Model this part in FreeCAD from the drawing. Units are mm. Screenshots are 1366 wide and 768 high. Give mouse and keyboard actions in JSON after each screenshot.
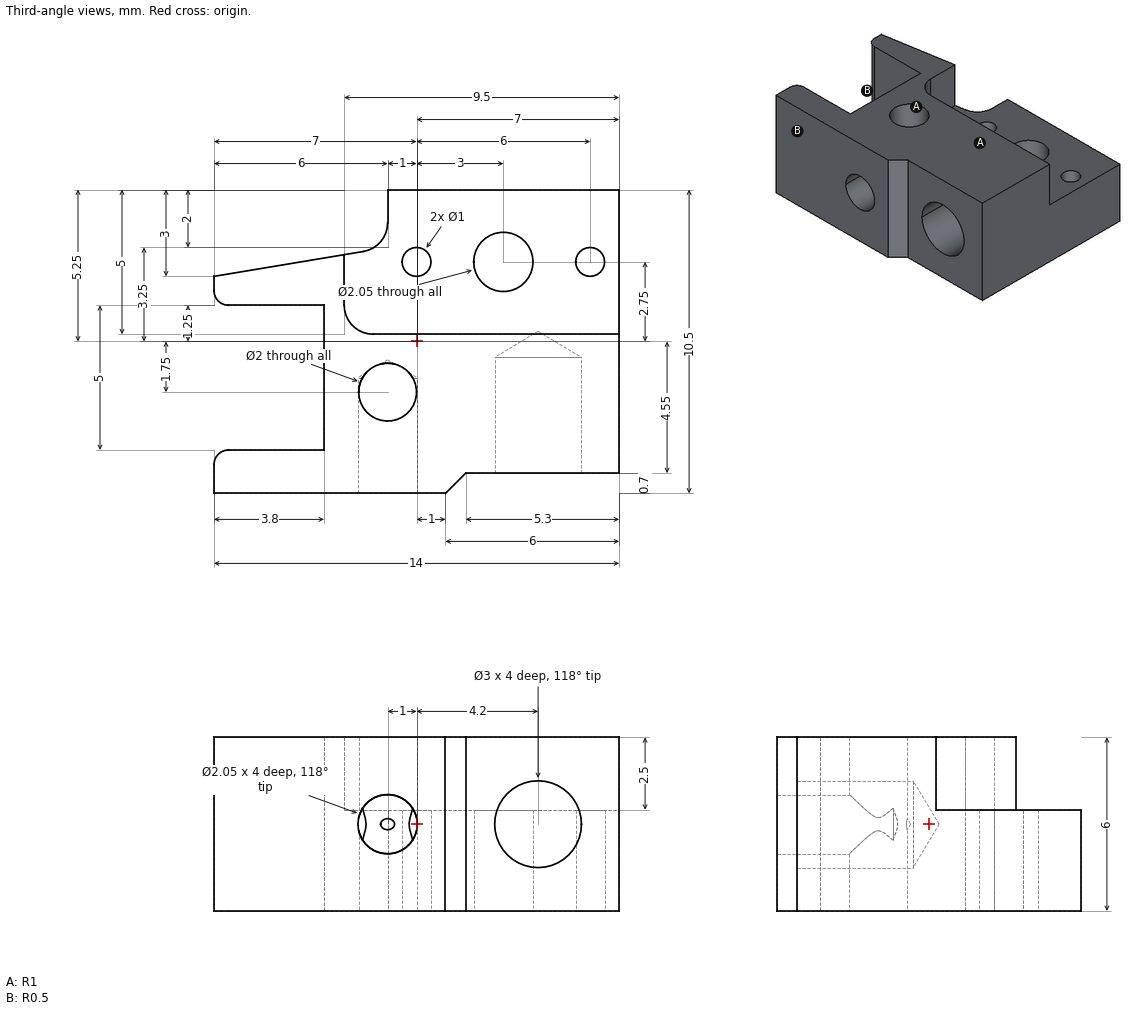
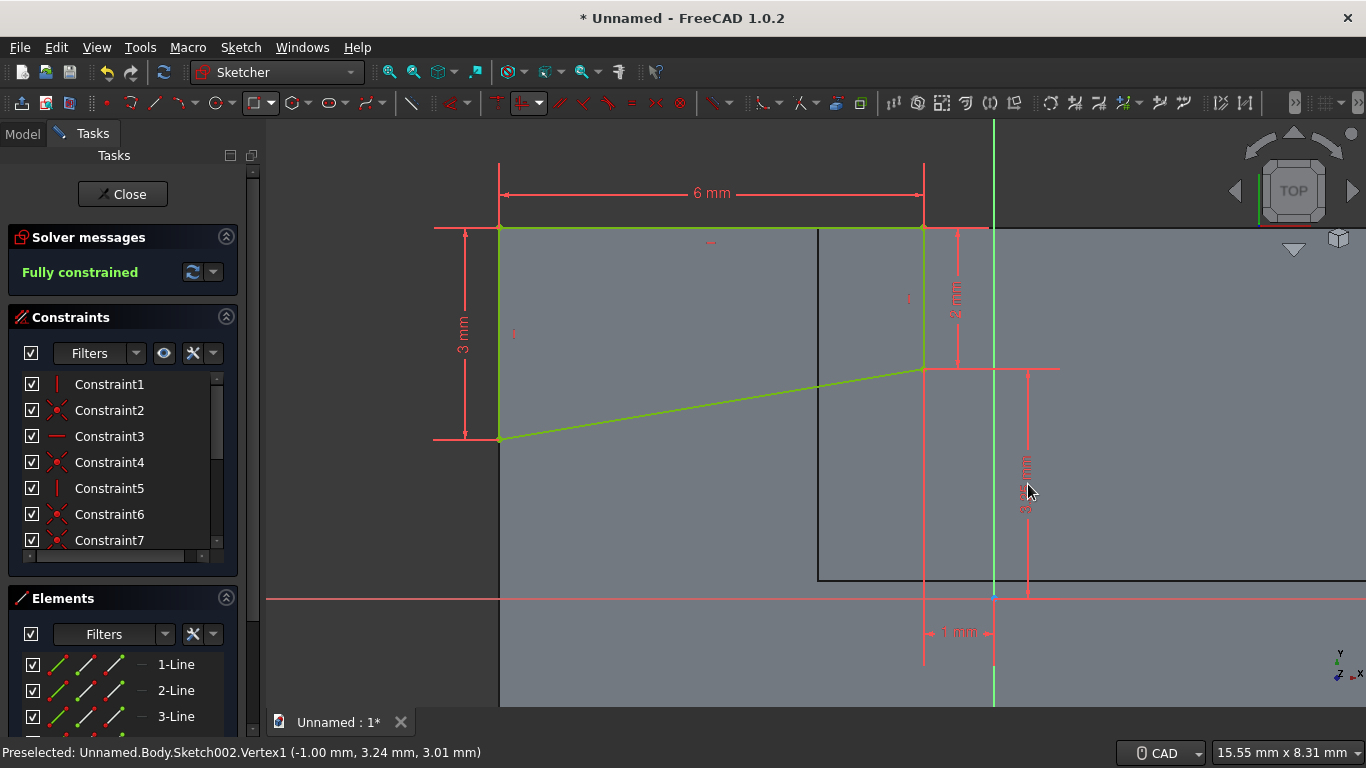
{"action": "left_click", "coordinate": [123, 194]}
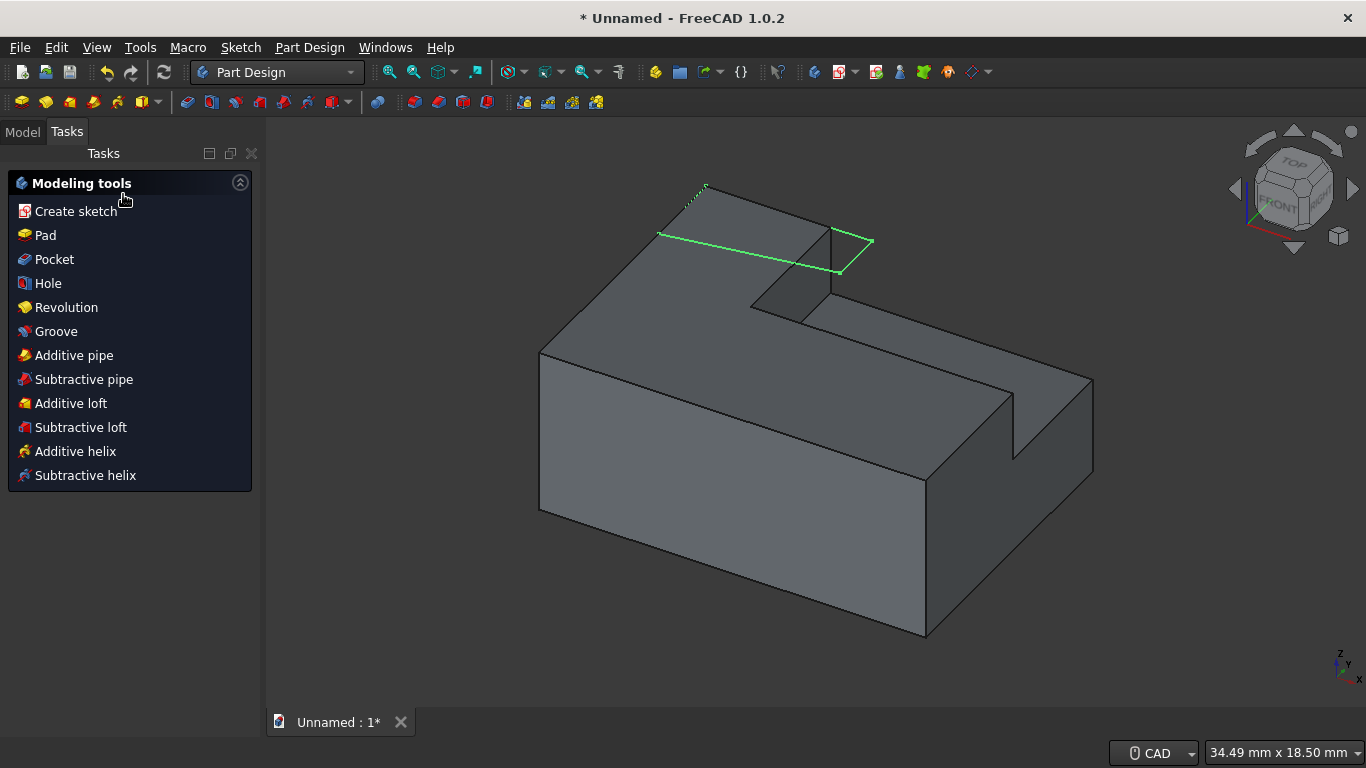
{"action": "left_click", "coordinate": [188, 102]}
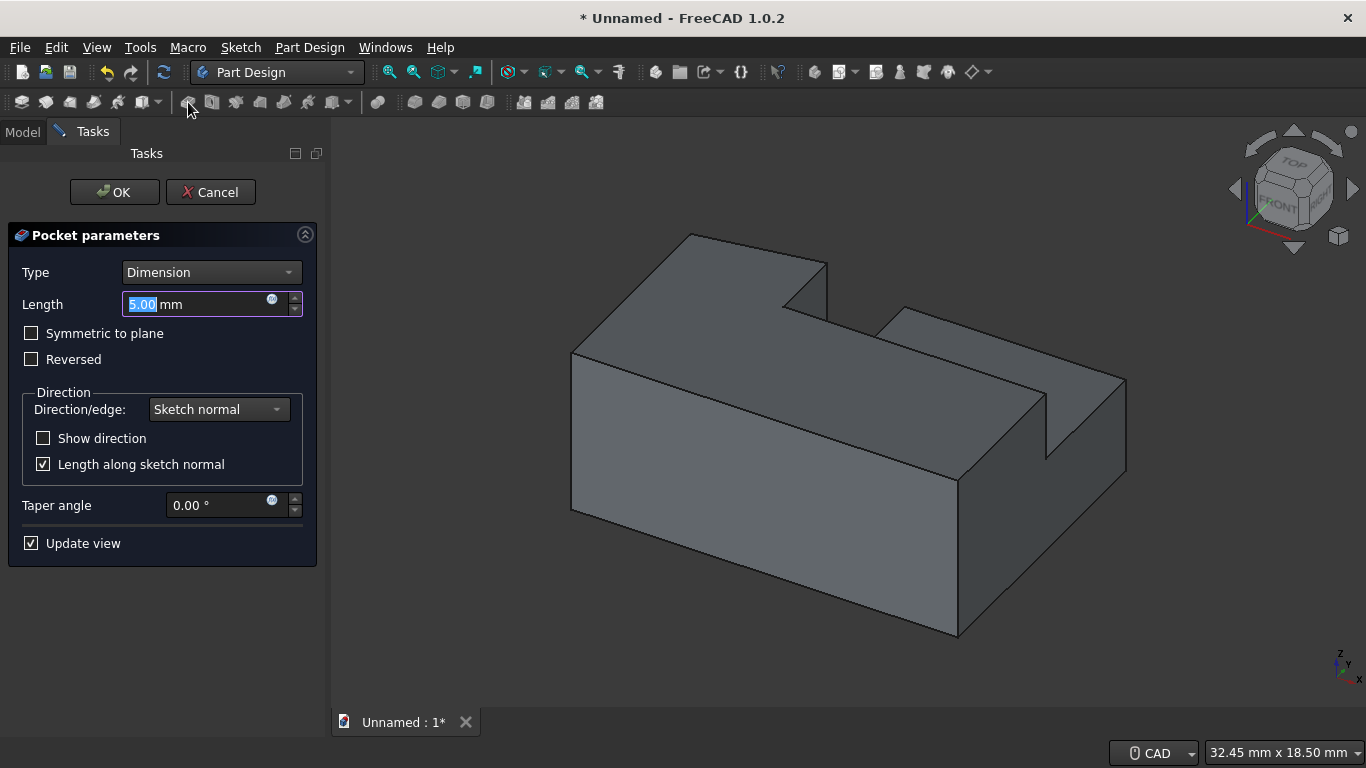
{"action": "left_click", "coordinate": [212, 272]}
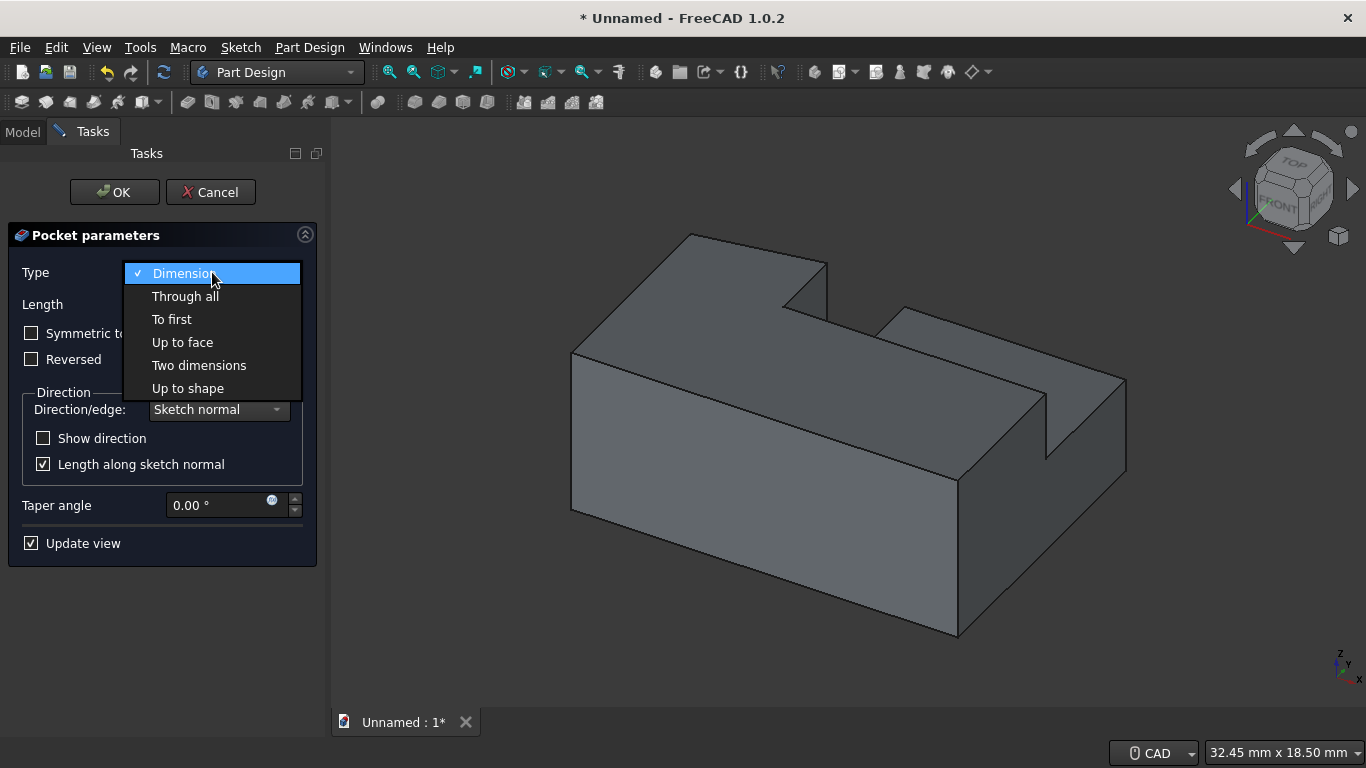
{"action": "left_click", "coordinate": [212, 296]}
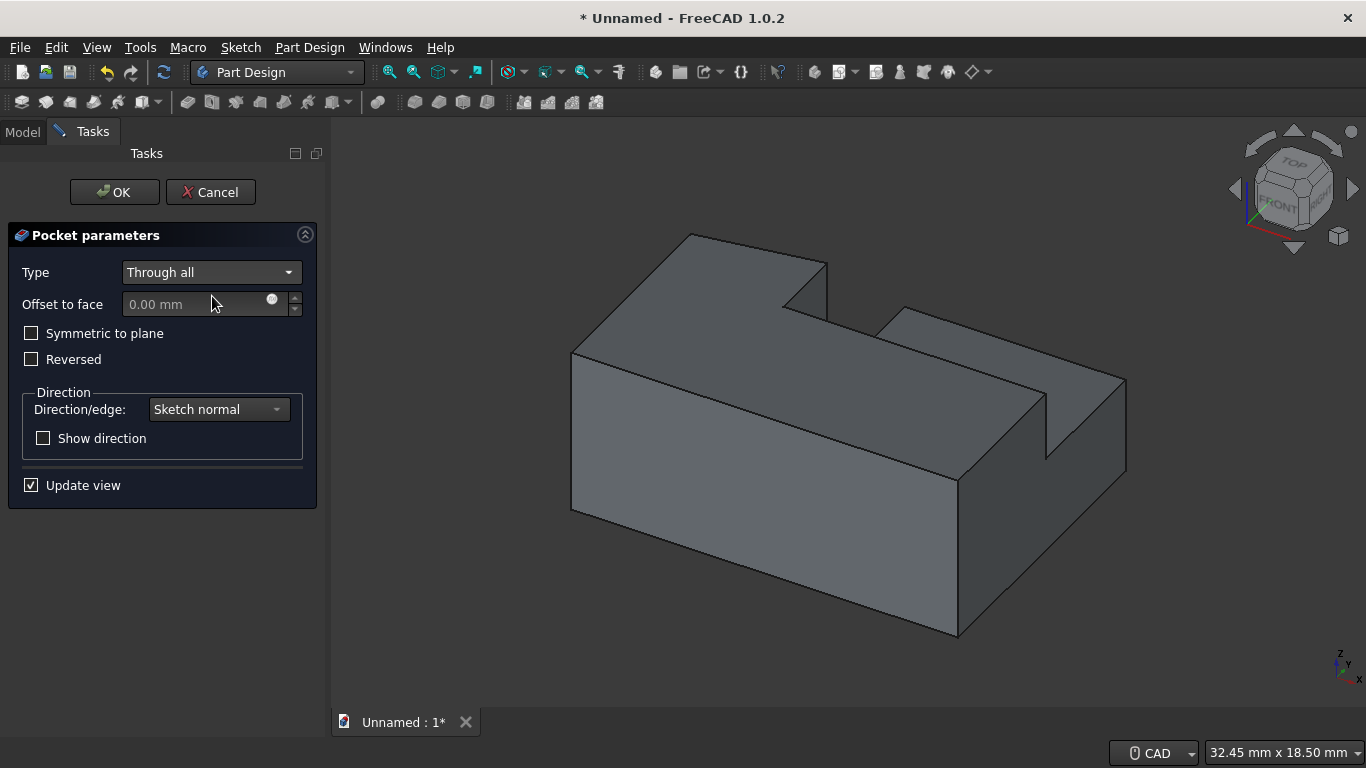
{"action": "left_click", "coordinate": [115, 192]}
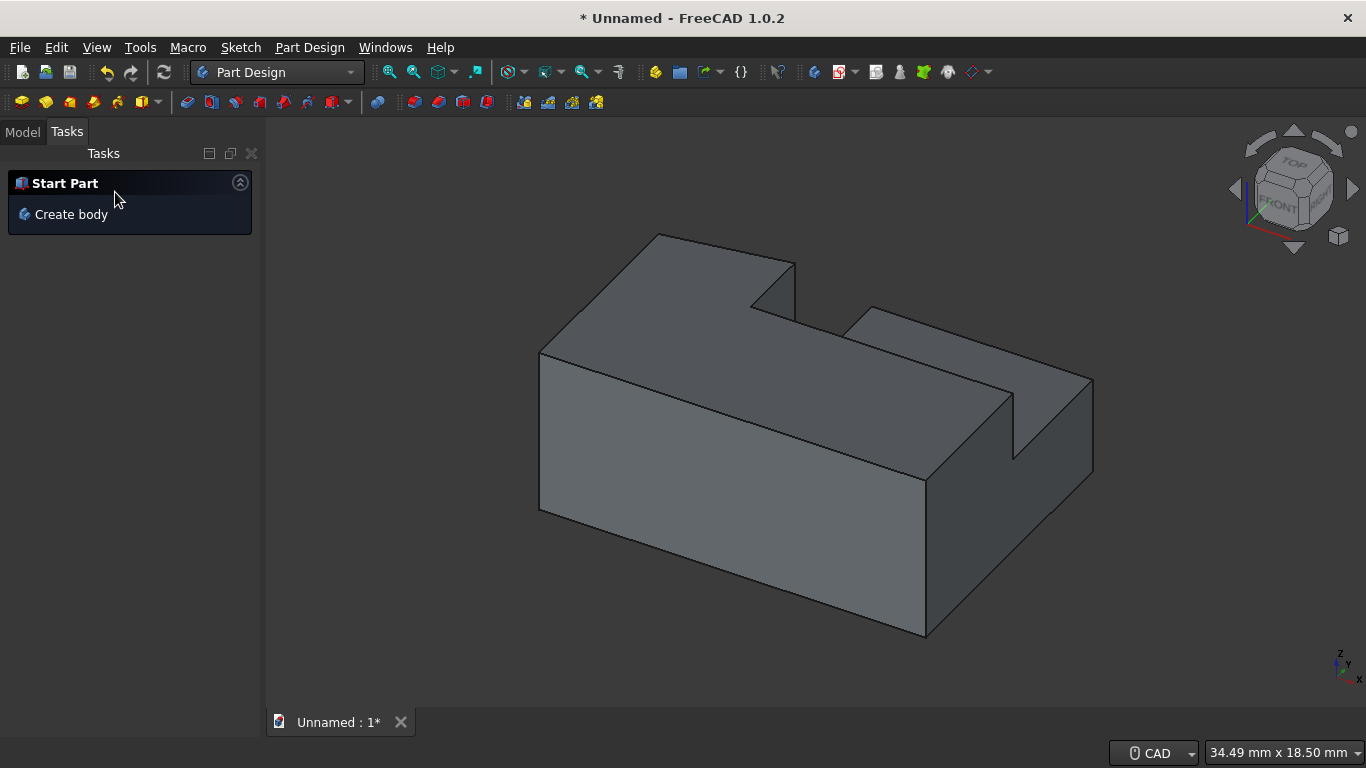
{"action": "key", "text": "0"}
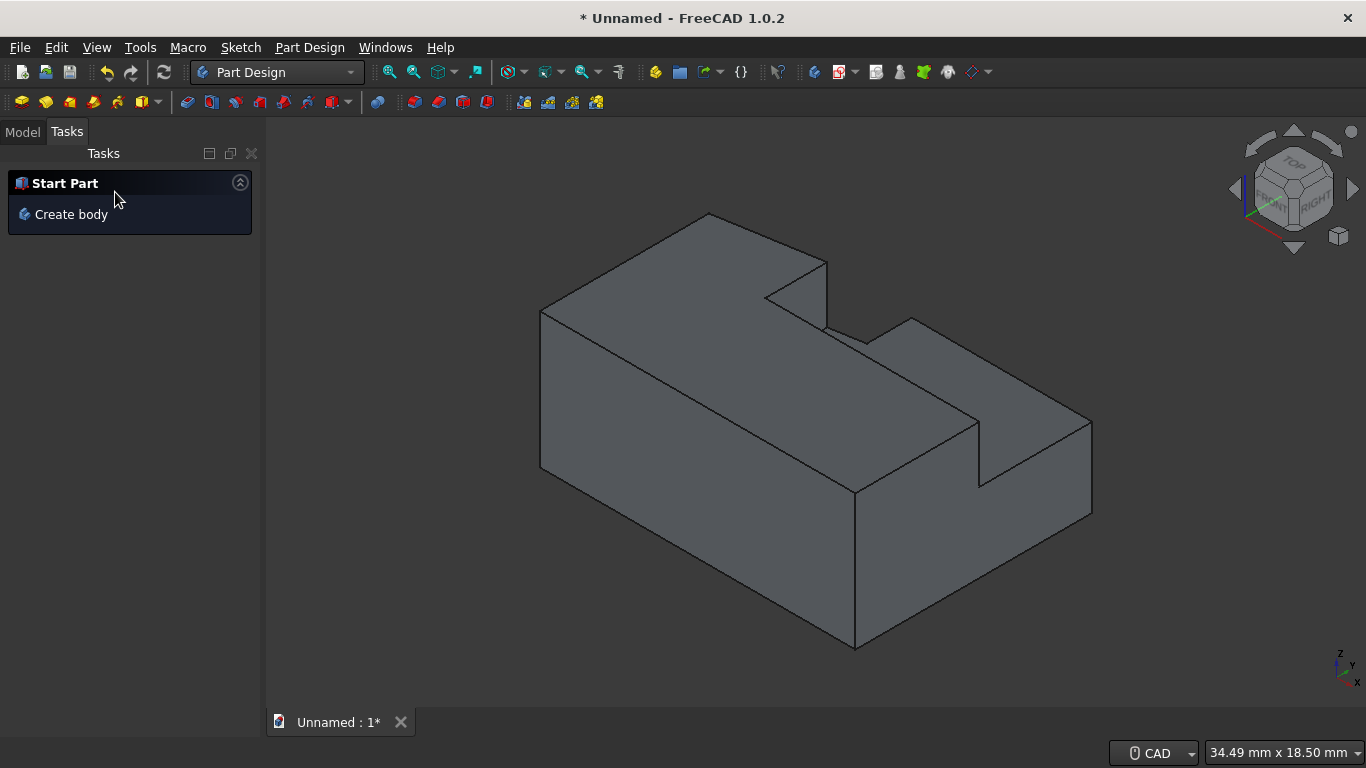
{"action": "key", "text": "2"}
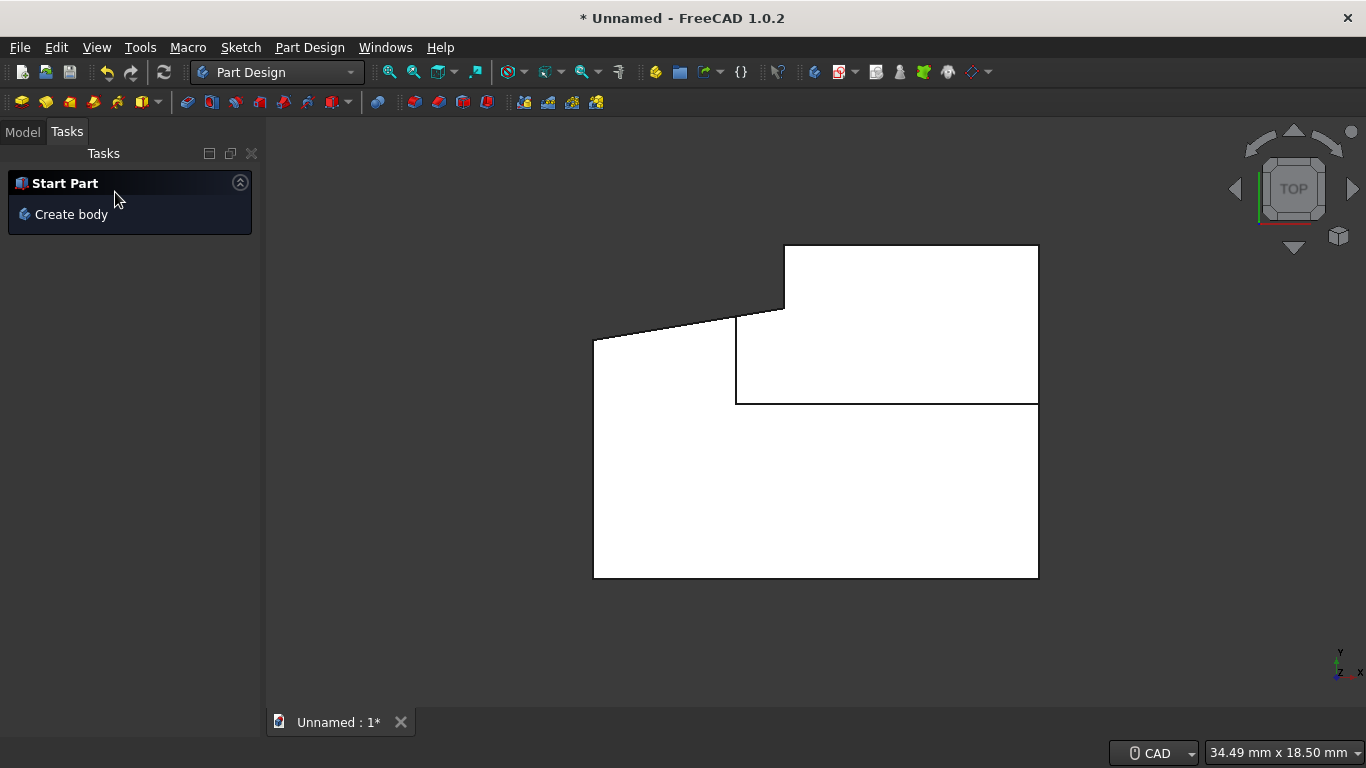
{"action": "key", "text": "1"}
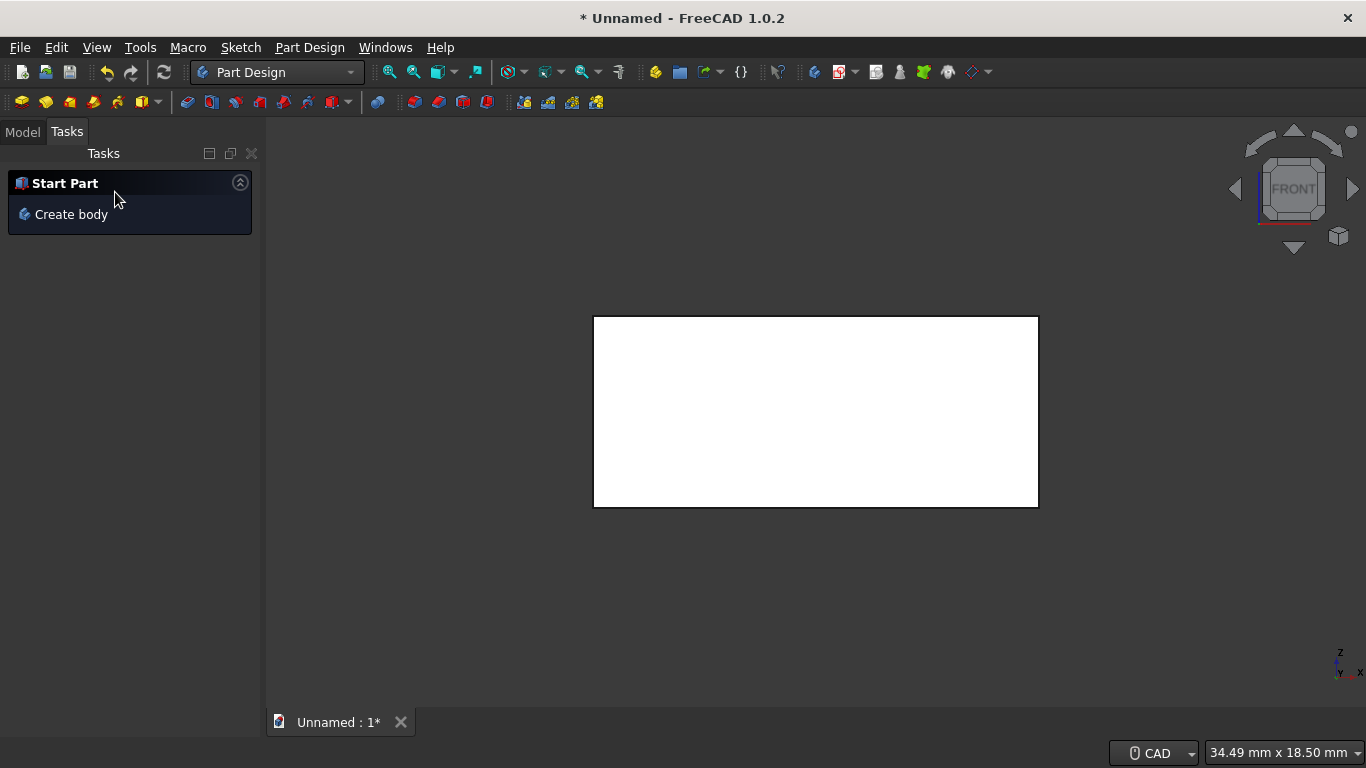
{"action": "left_click", "coordinate": [390, 72]}